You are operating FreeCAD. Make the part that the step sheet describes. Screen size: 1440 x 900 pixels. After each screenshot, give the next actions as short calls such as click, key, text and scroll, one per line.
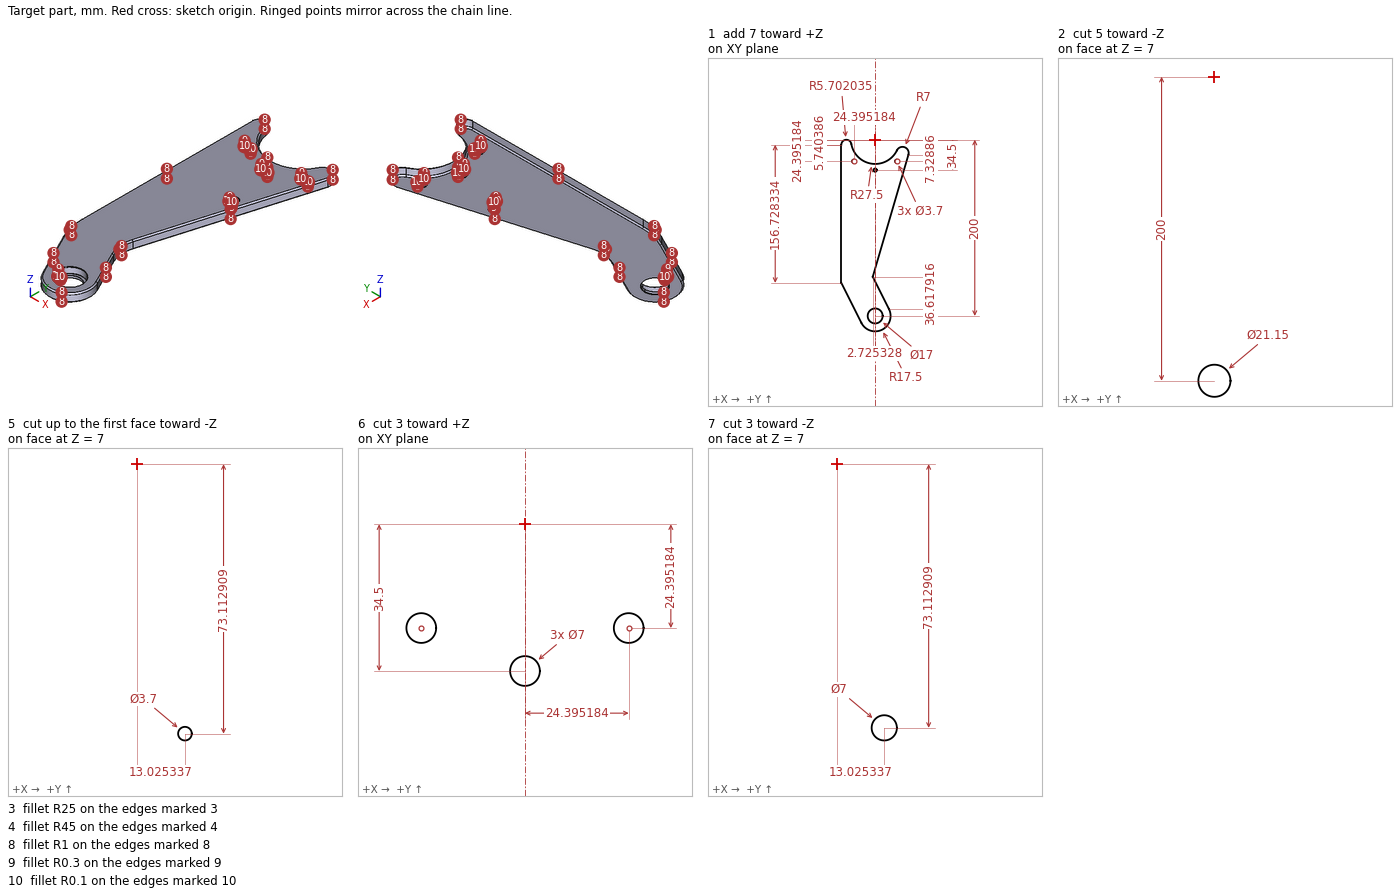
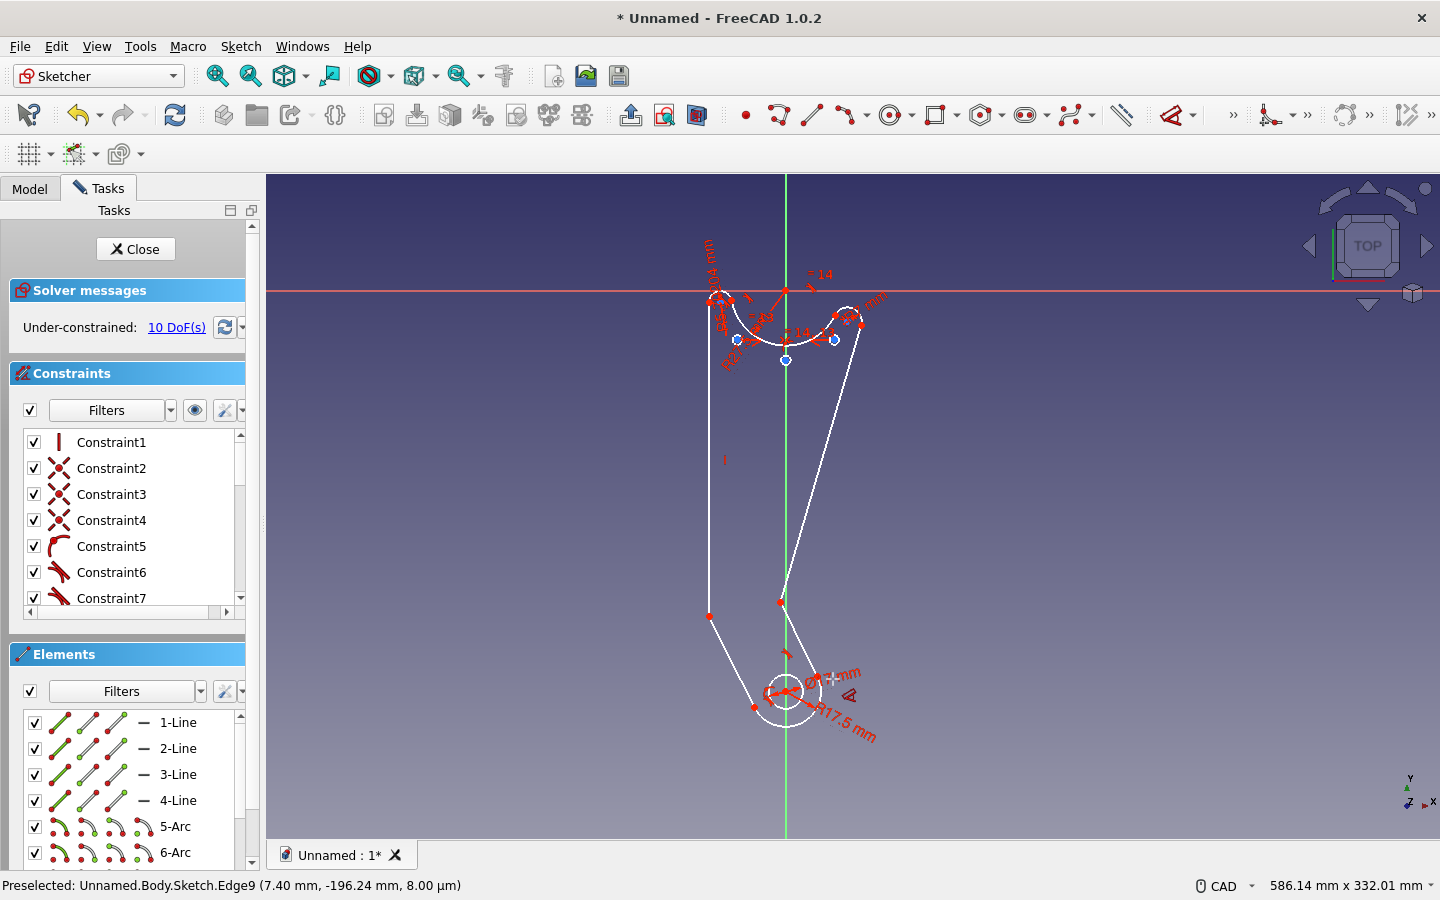
scroll(738, 335, up, 9)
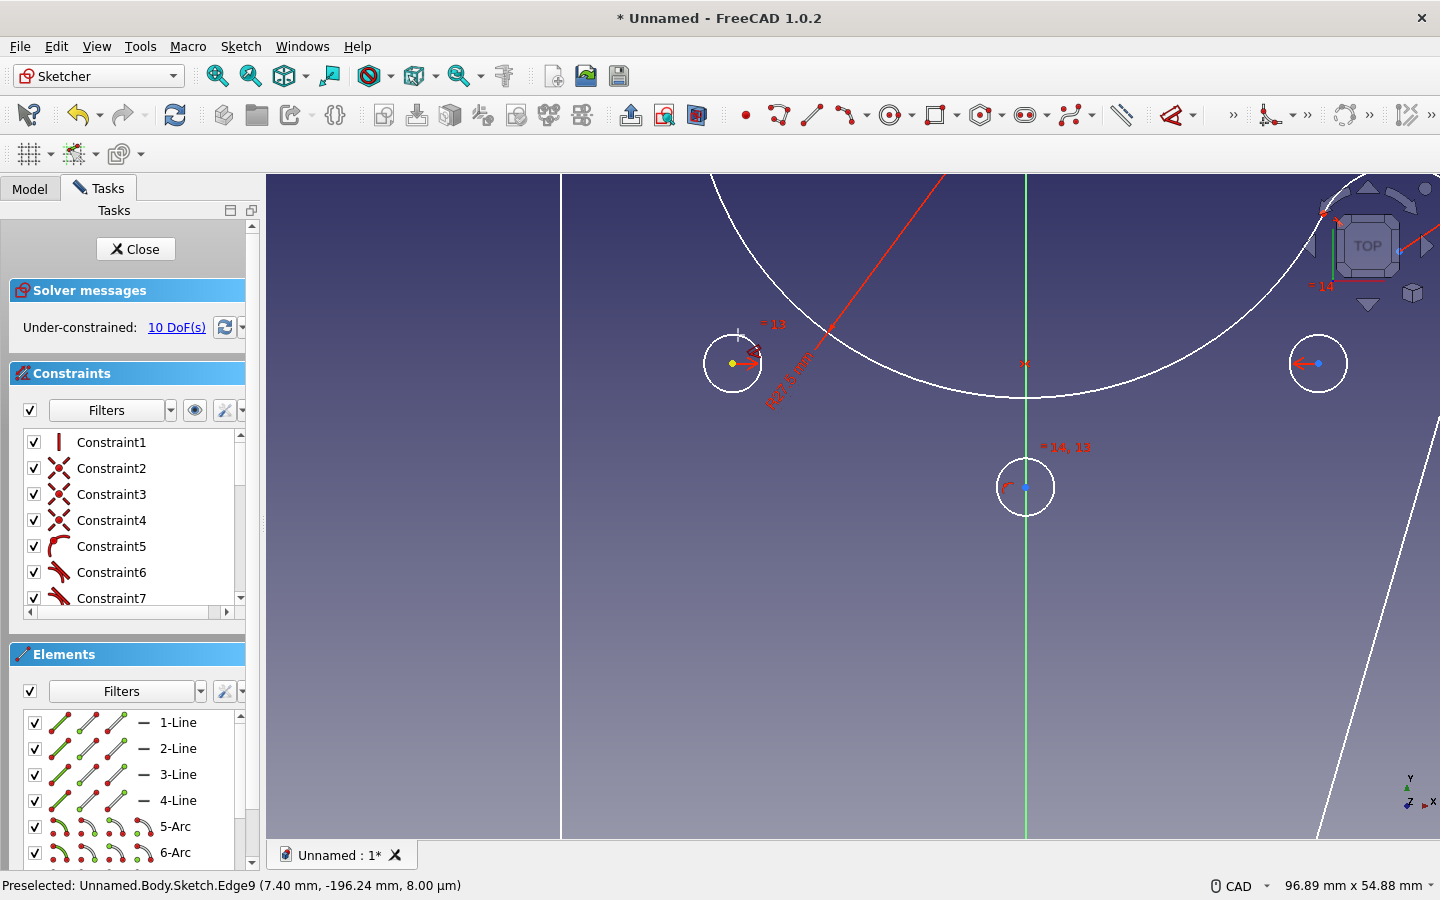
click(734, 335)
click(735, 303)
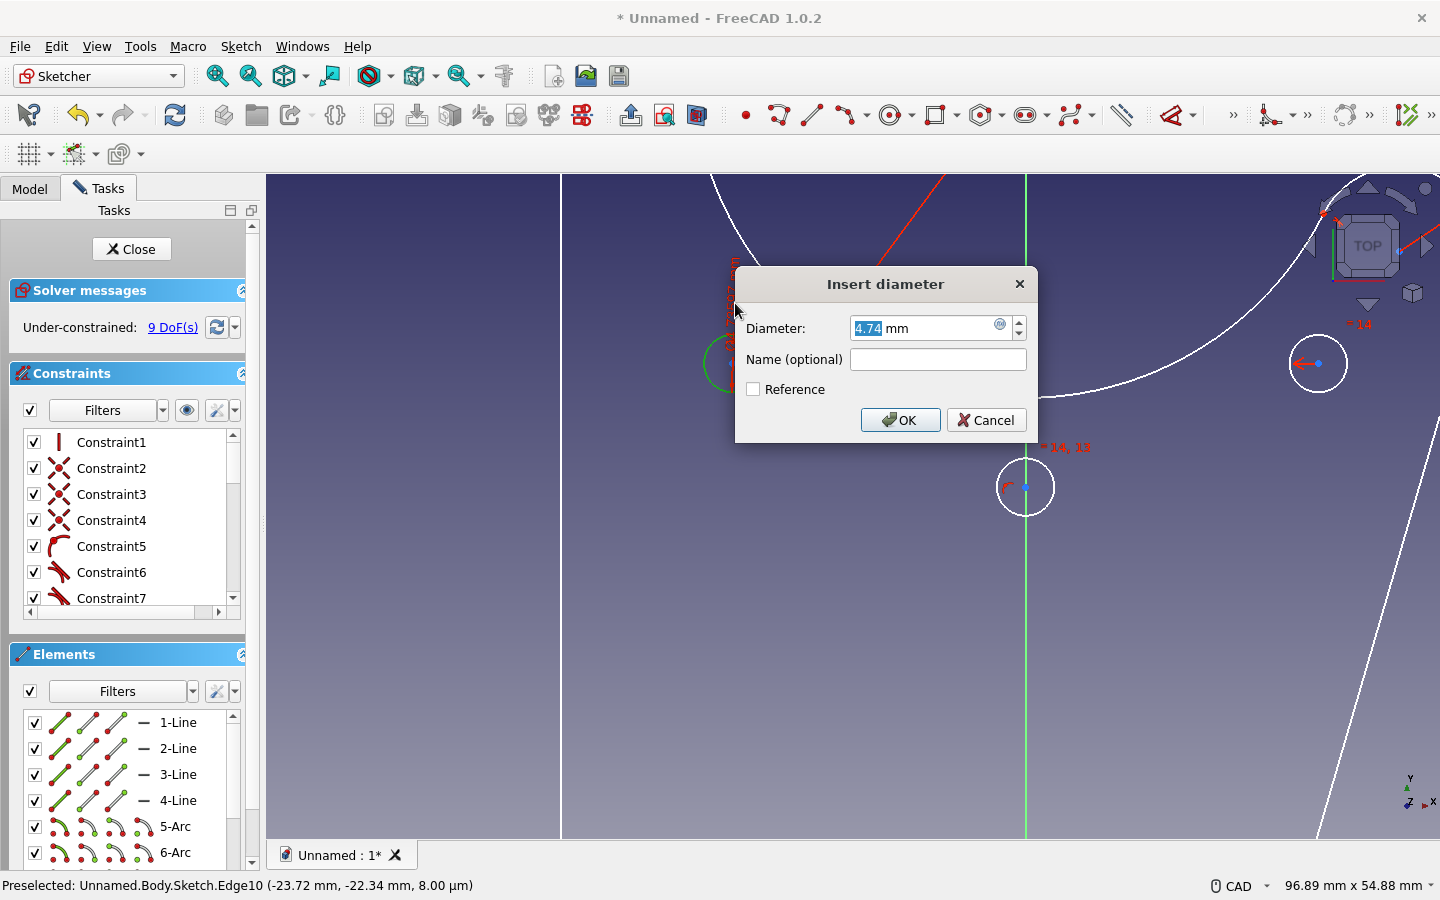
text(3.7)
key(Return)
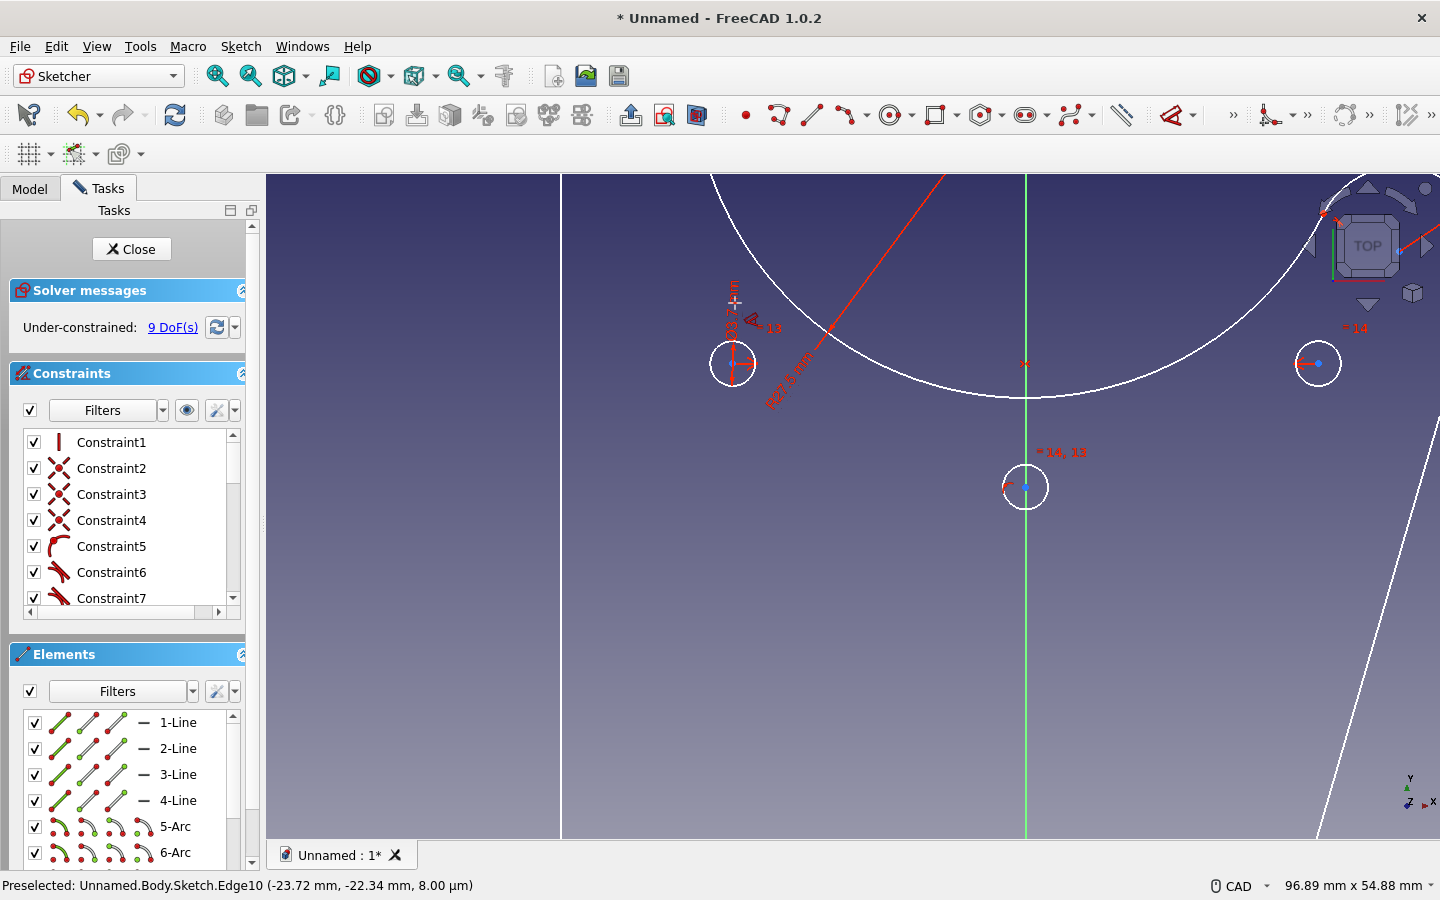
scroll(738, 335, down, 9)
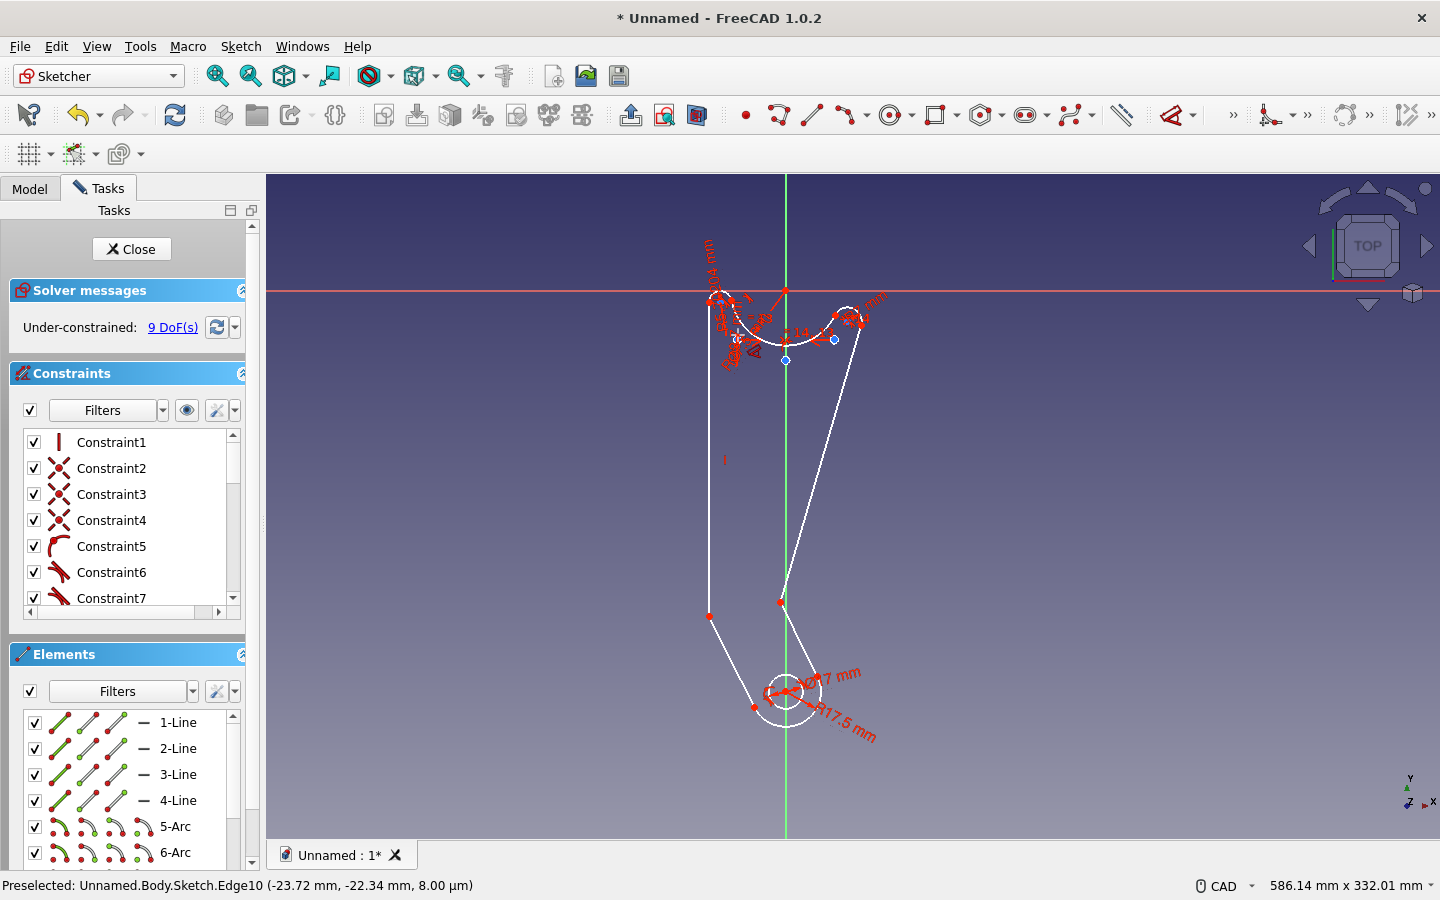
click(786, 692)
click(820, 399)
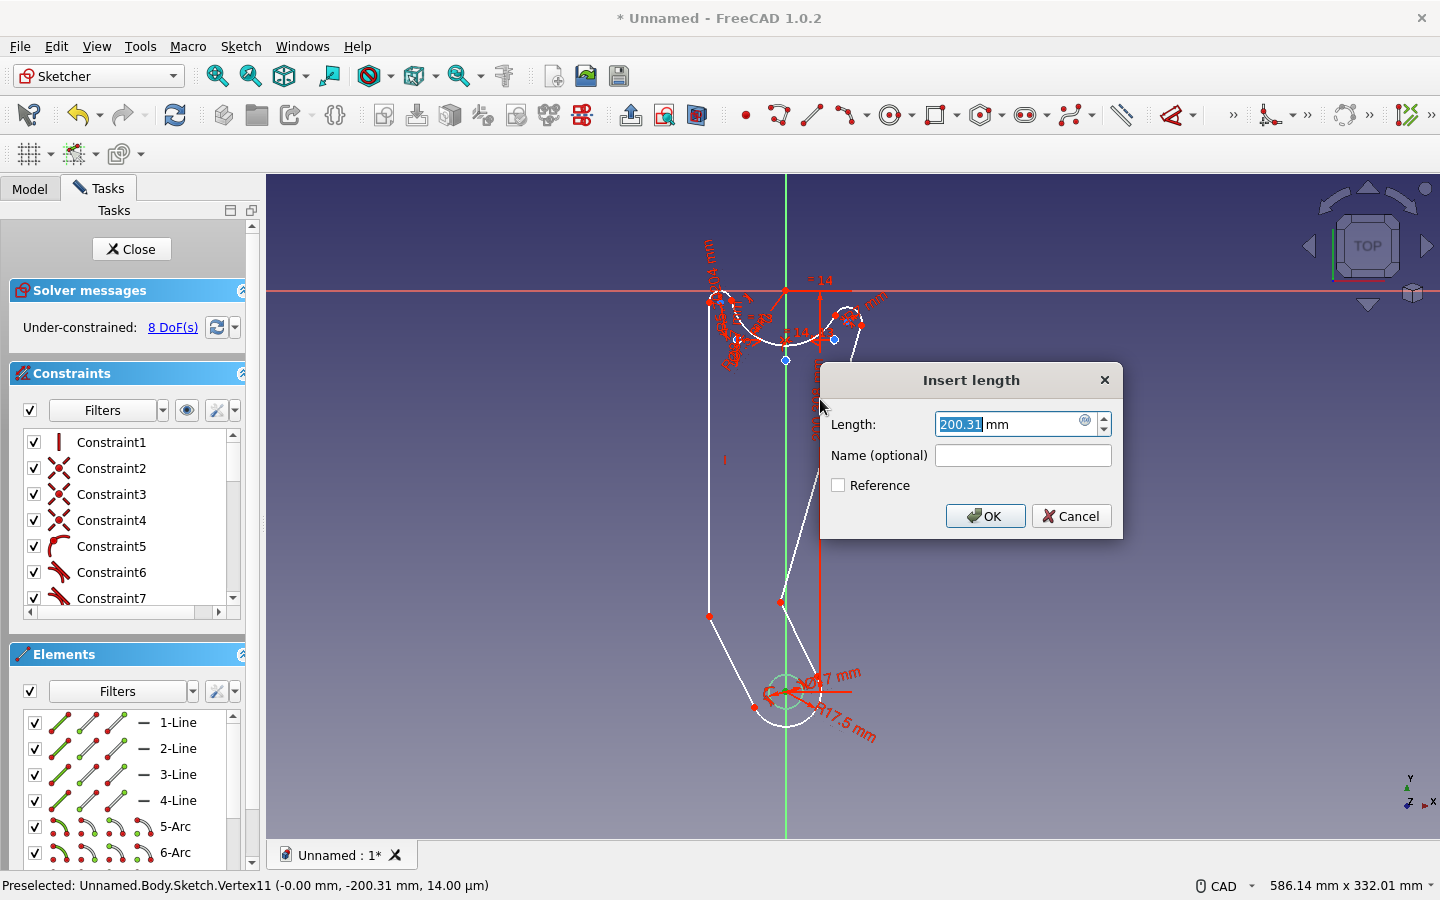
text(200)
key(Return)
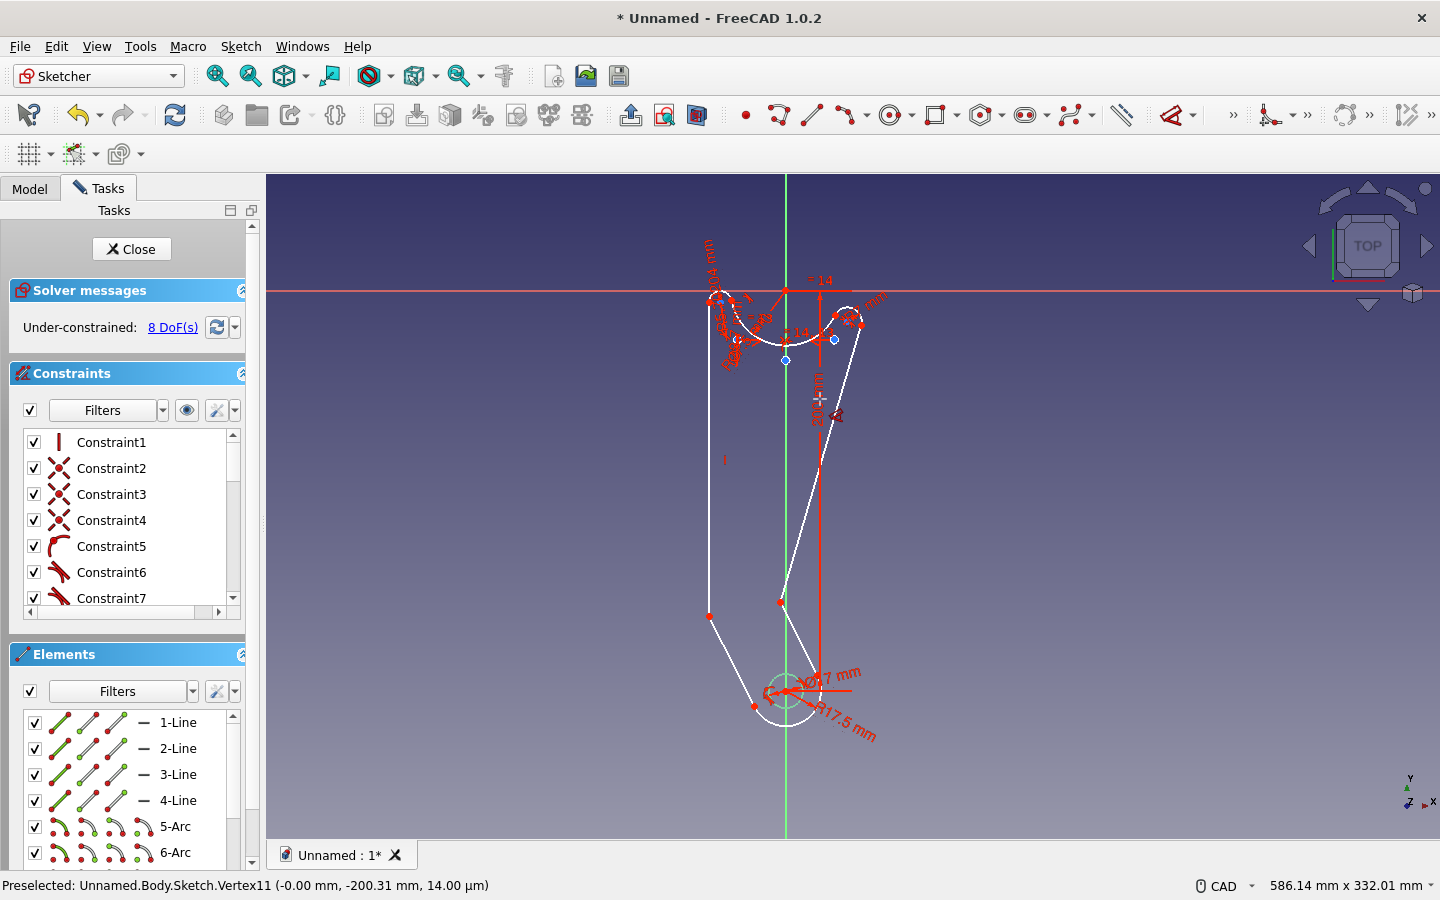
click(786, 360)
click(820, 350)